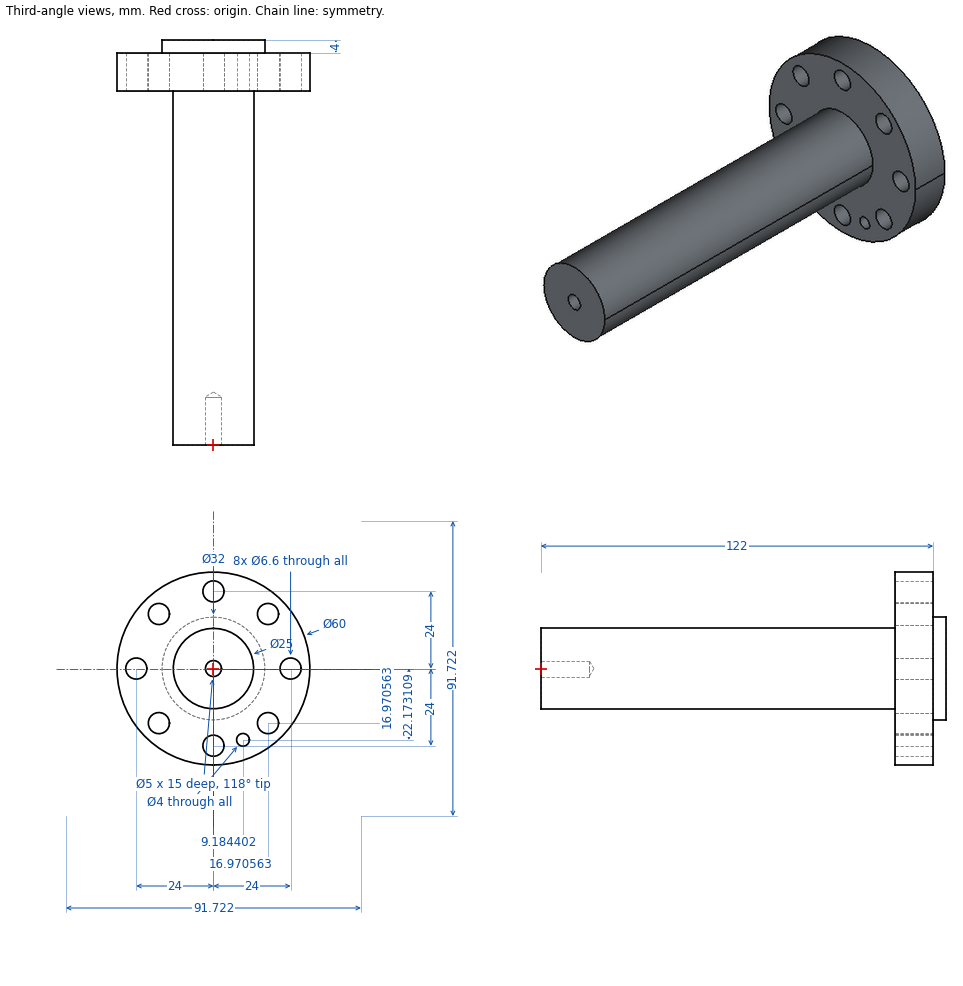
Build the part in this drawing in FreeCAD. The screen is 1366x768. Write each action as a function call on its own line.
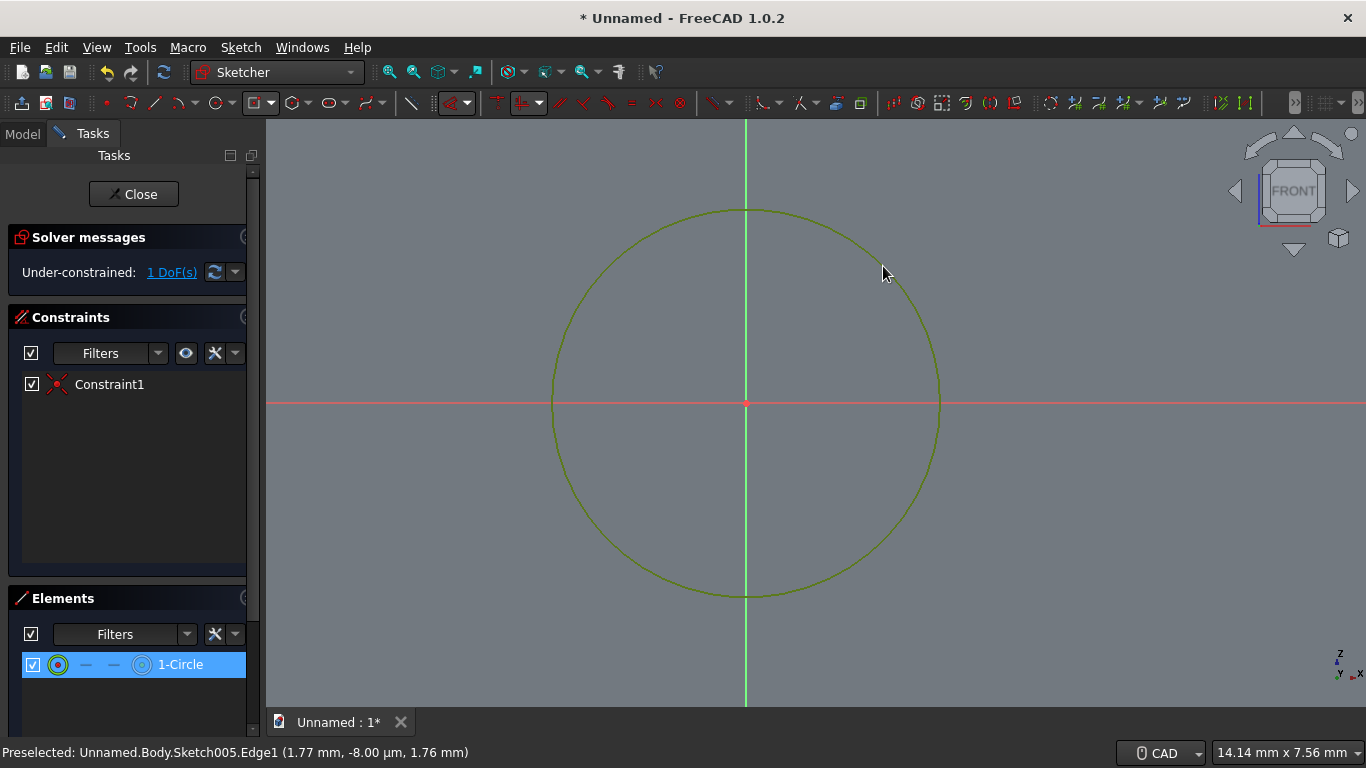
click(470, 104)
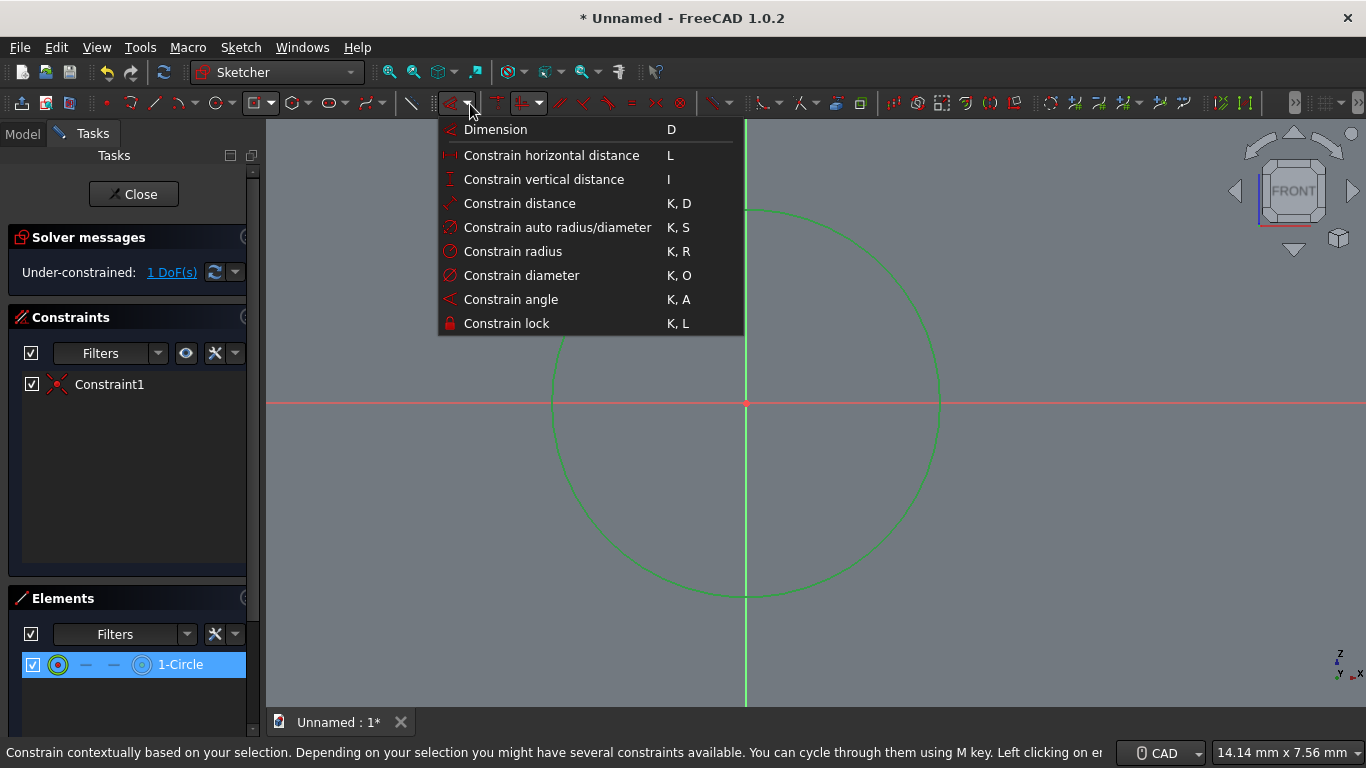
click(591, 275)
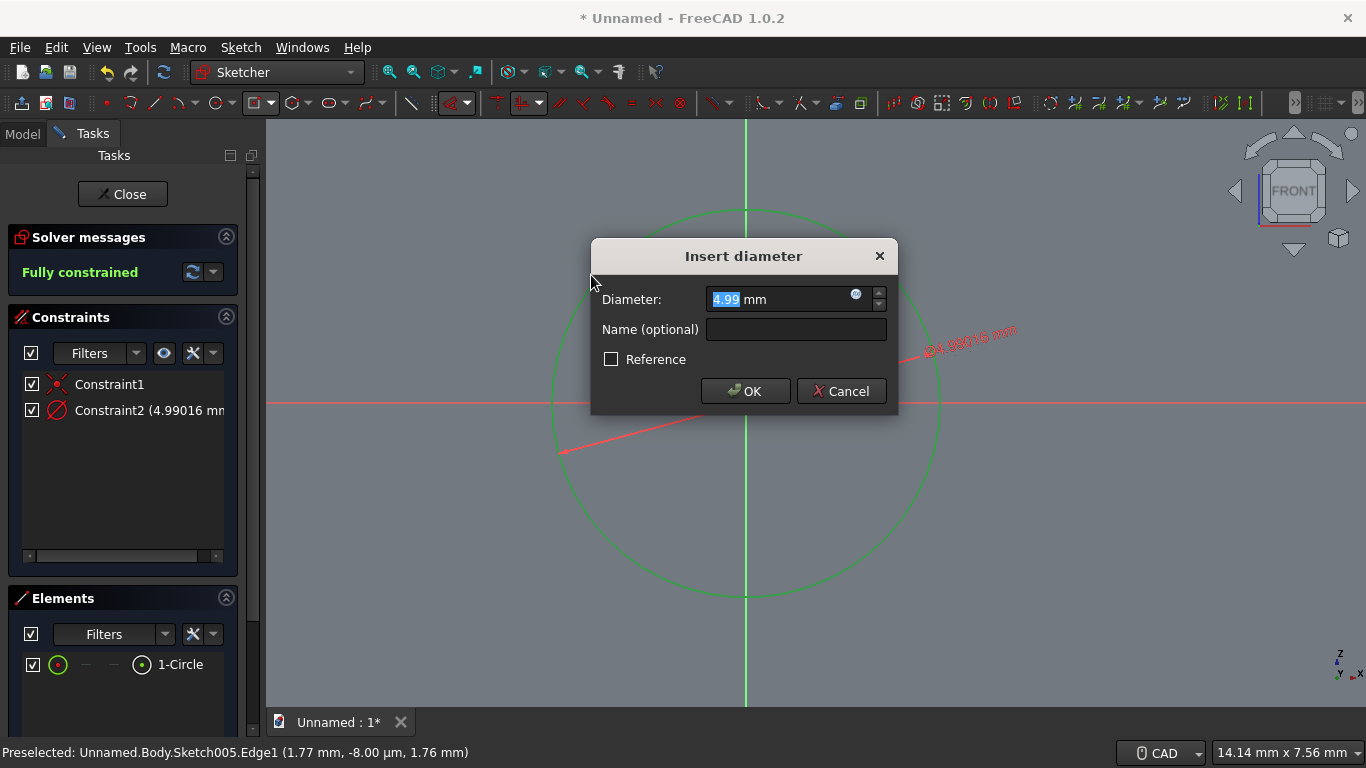
text(5)
key(Return)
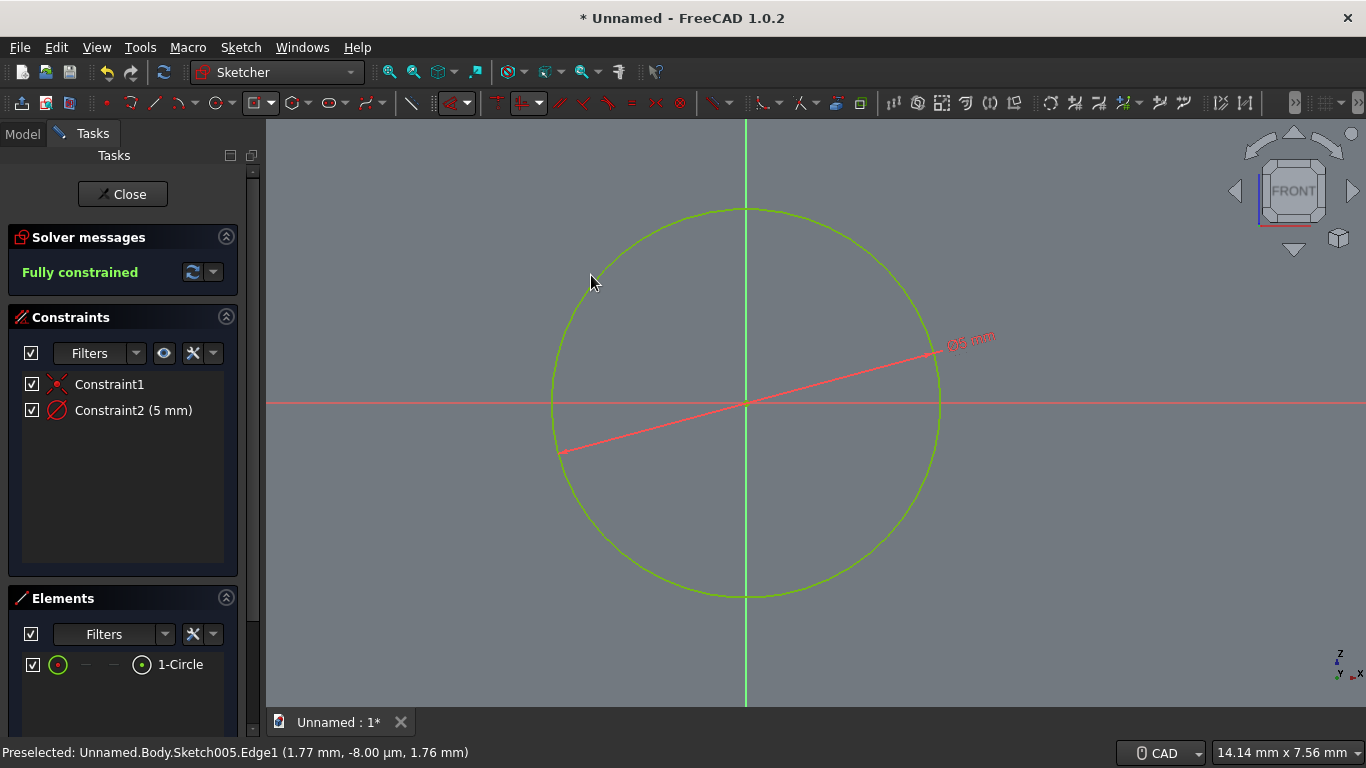
click(123, 194)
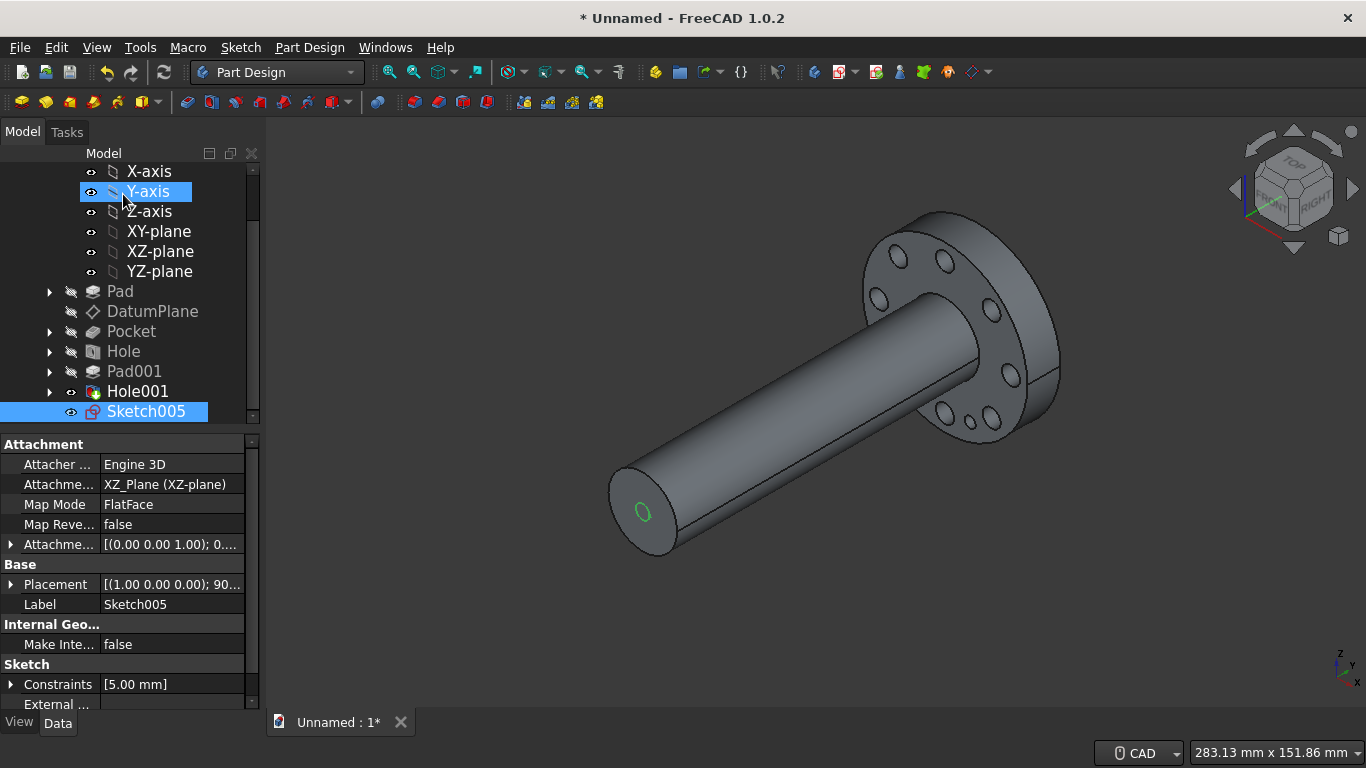
click(212, 102)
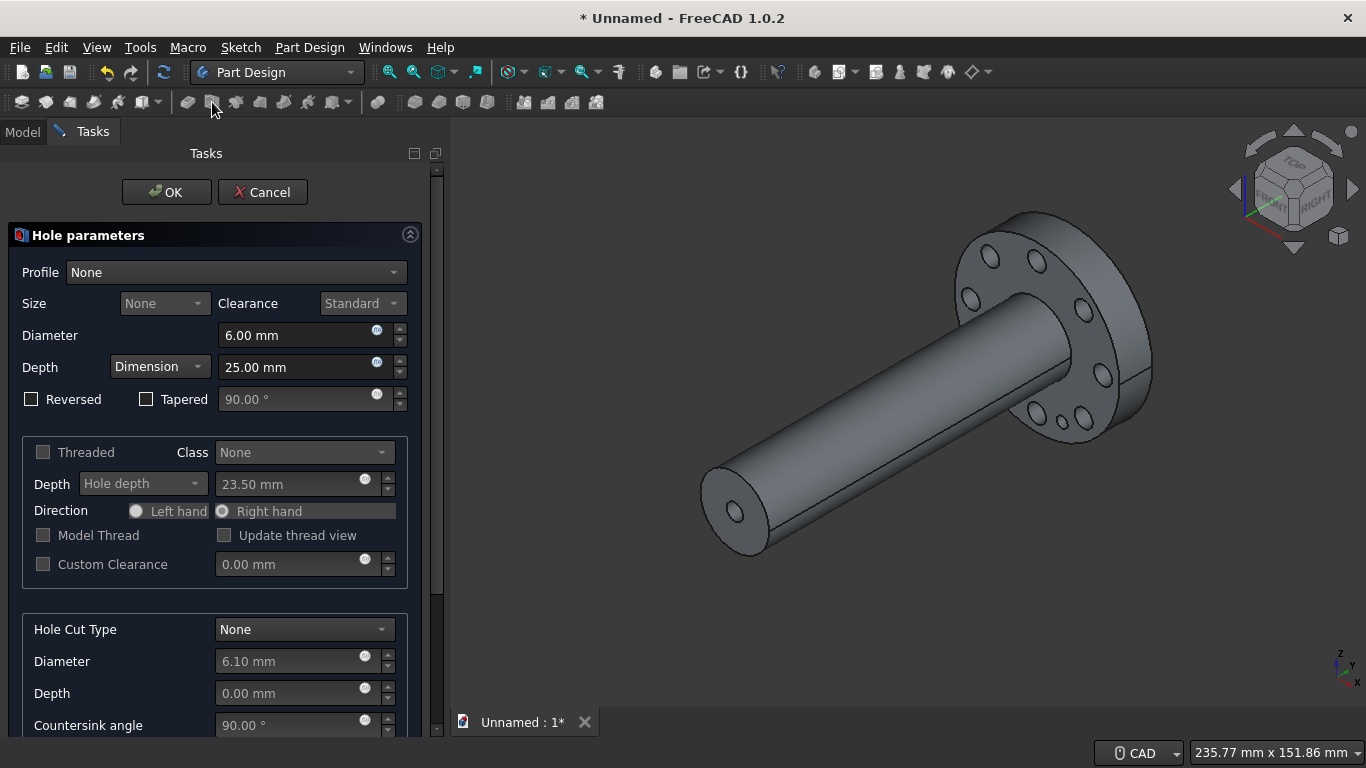
triple_click(305, 335)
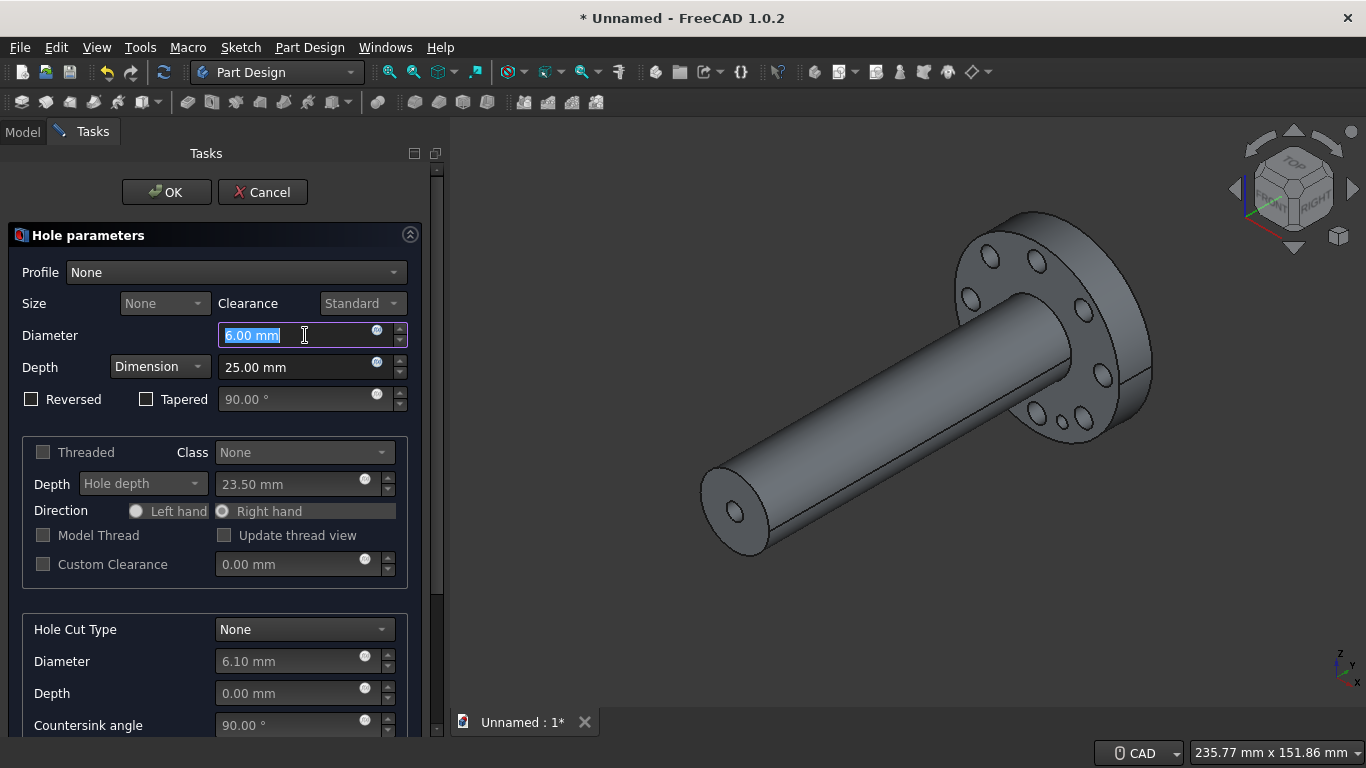
text(5)
key(Tab)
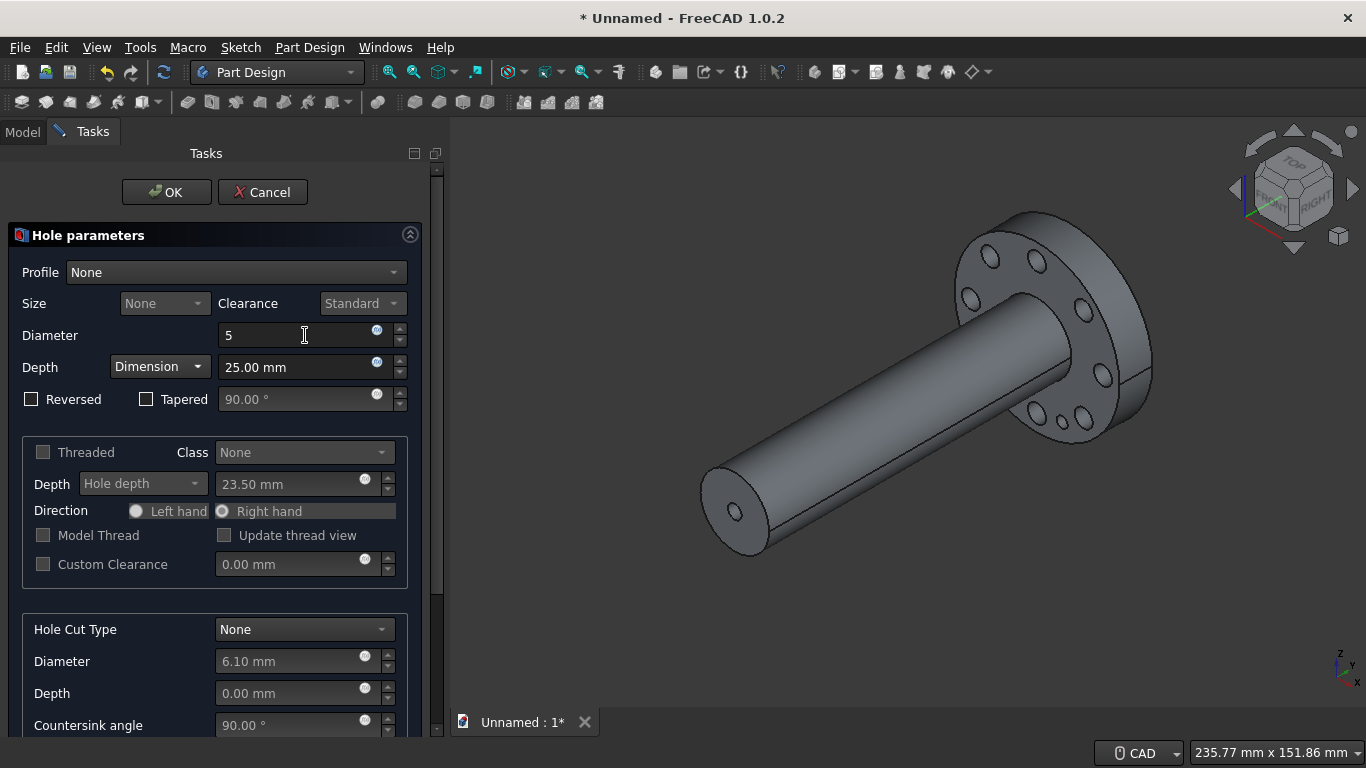
triple_click(305, 367)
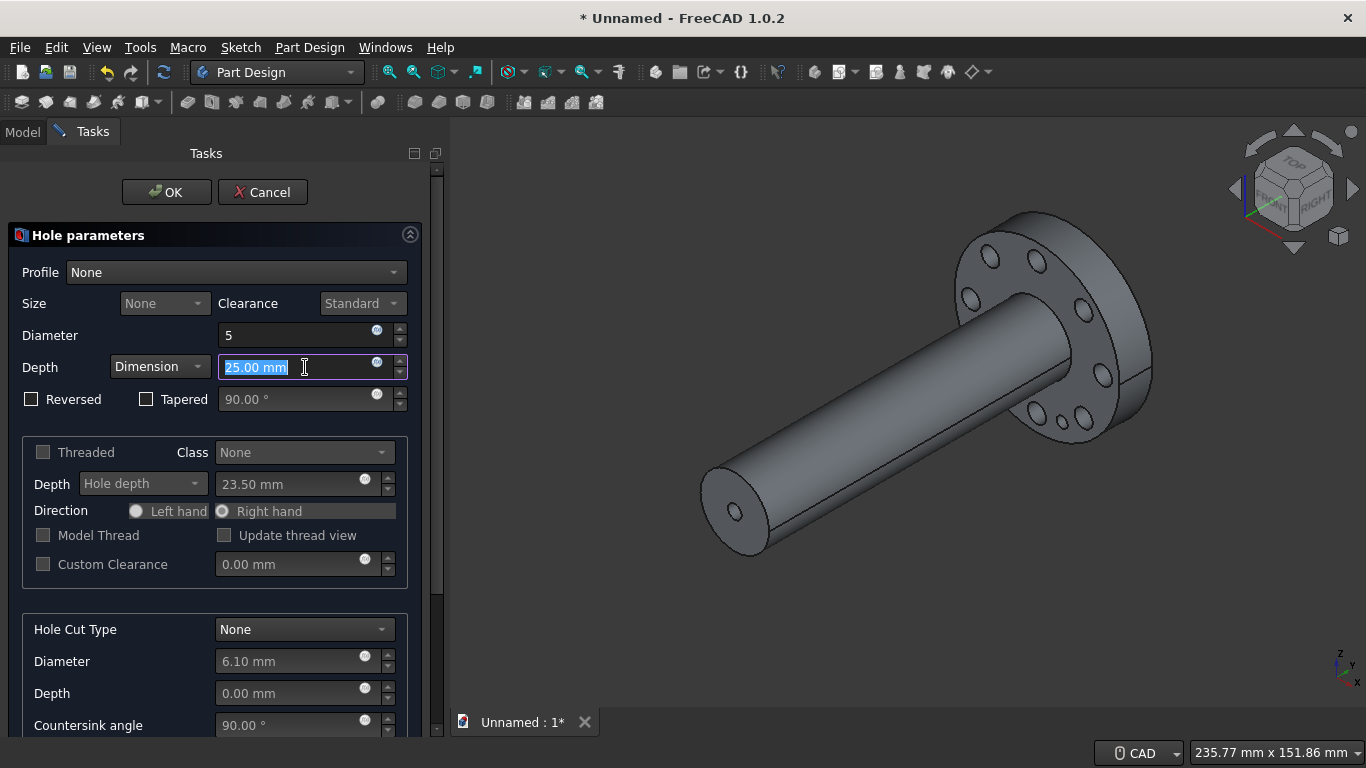
text(15)
key(Tab)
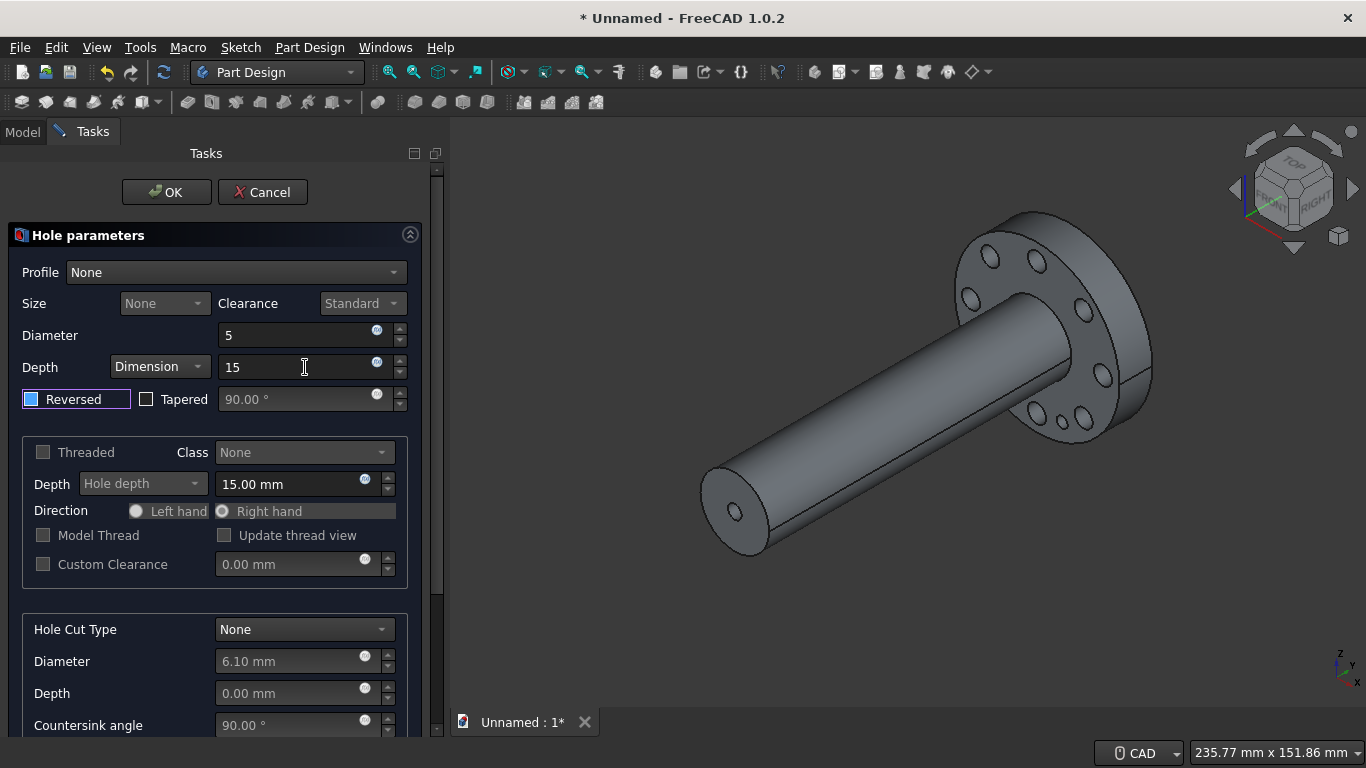
click(167, 192)